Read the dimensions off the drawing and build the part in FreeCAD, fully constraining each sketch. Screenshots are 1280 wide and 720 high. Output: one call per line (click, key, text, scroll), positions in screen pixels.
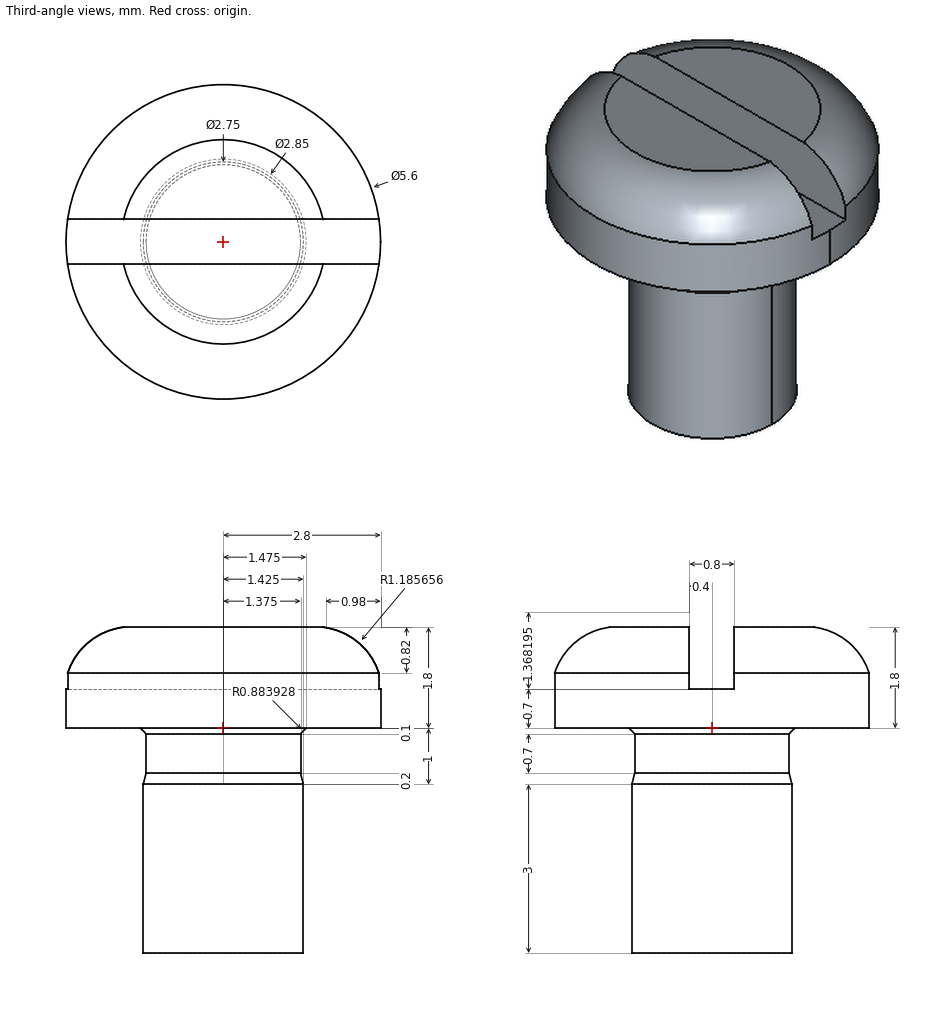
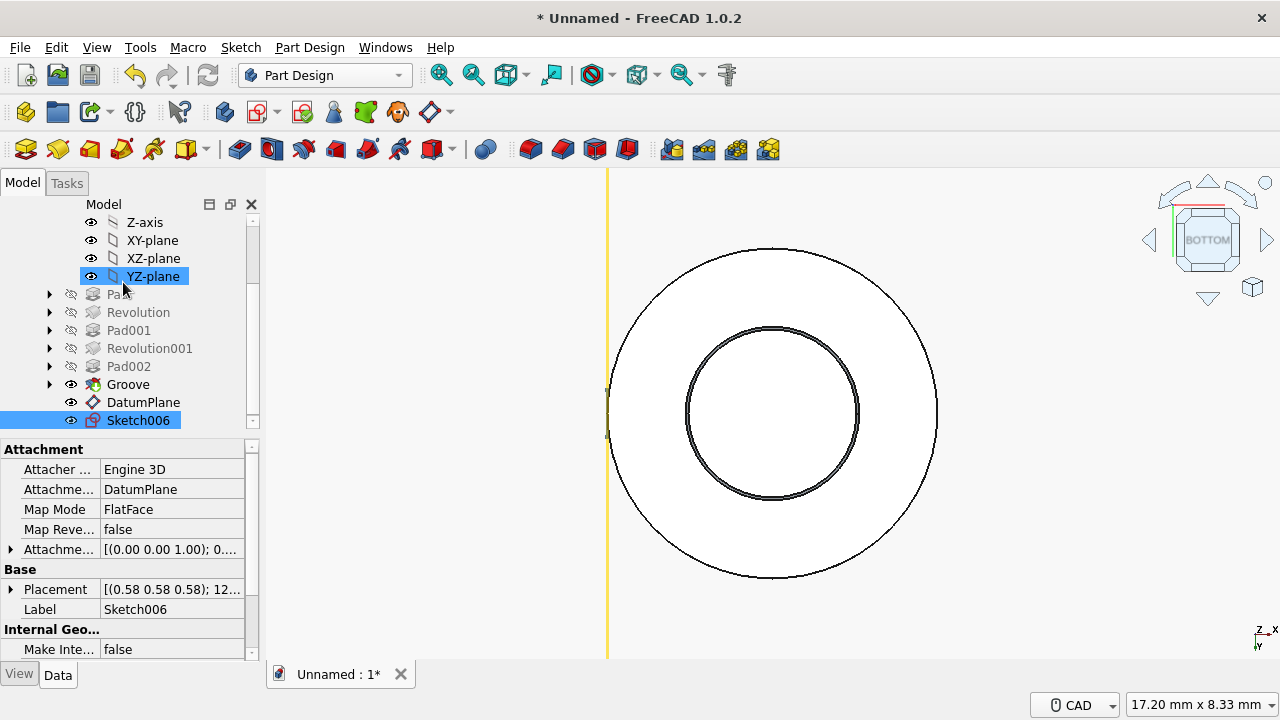
click(240, 150)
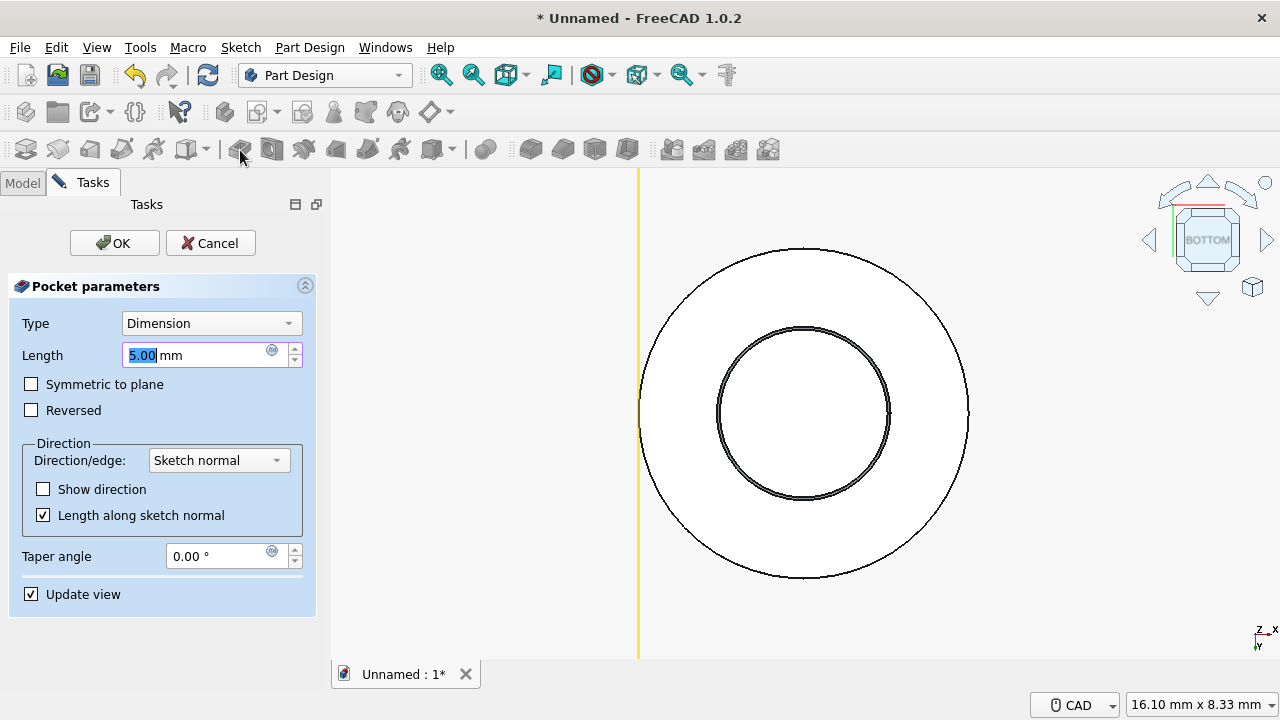
click(212, 324)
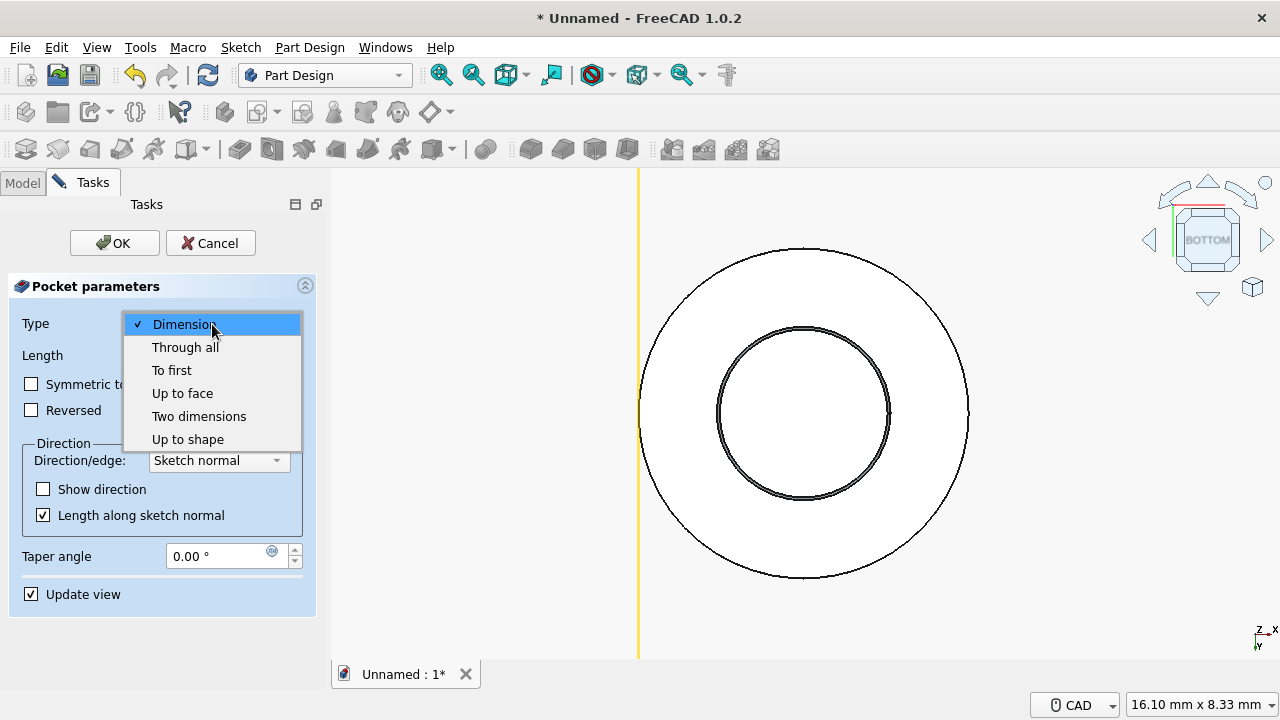
click(212, 348)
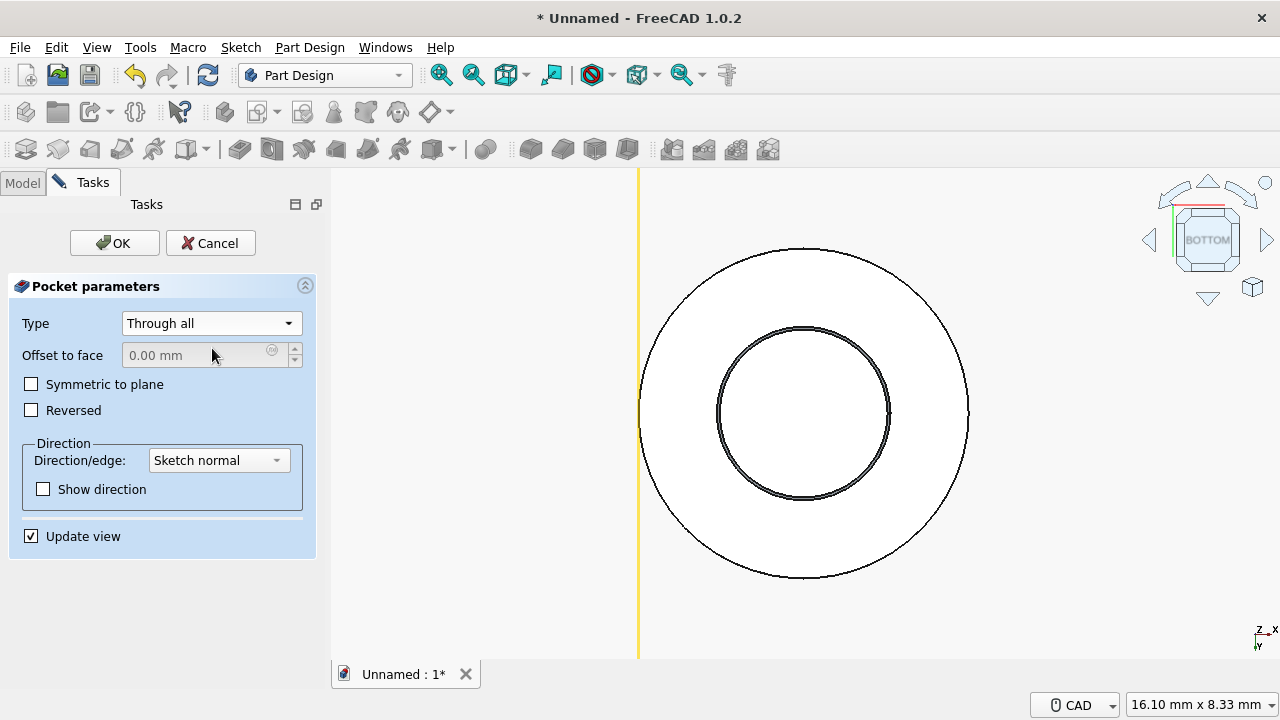
click(30, 410)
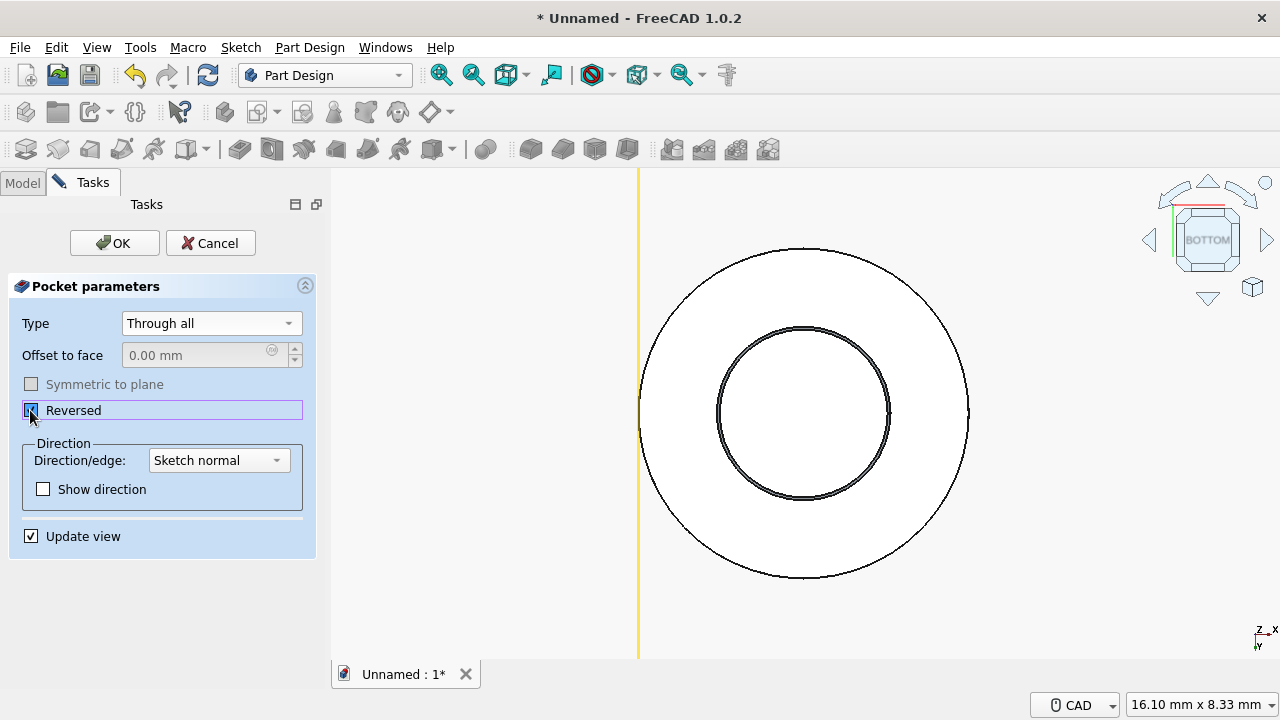
click(115, 243)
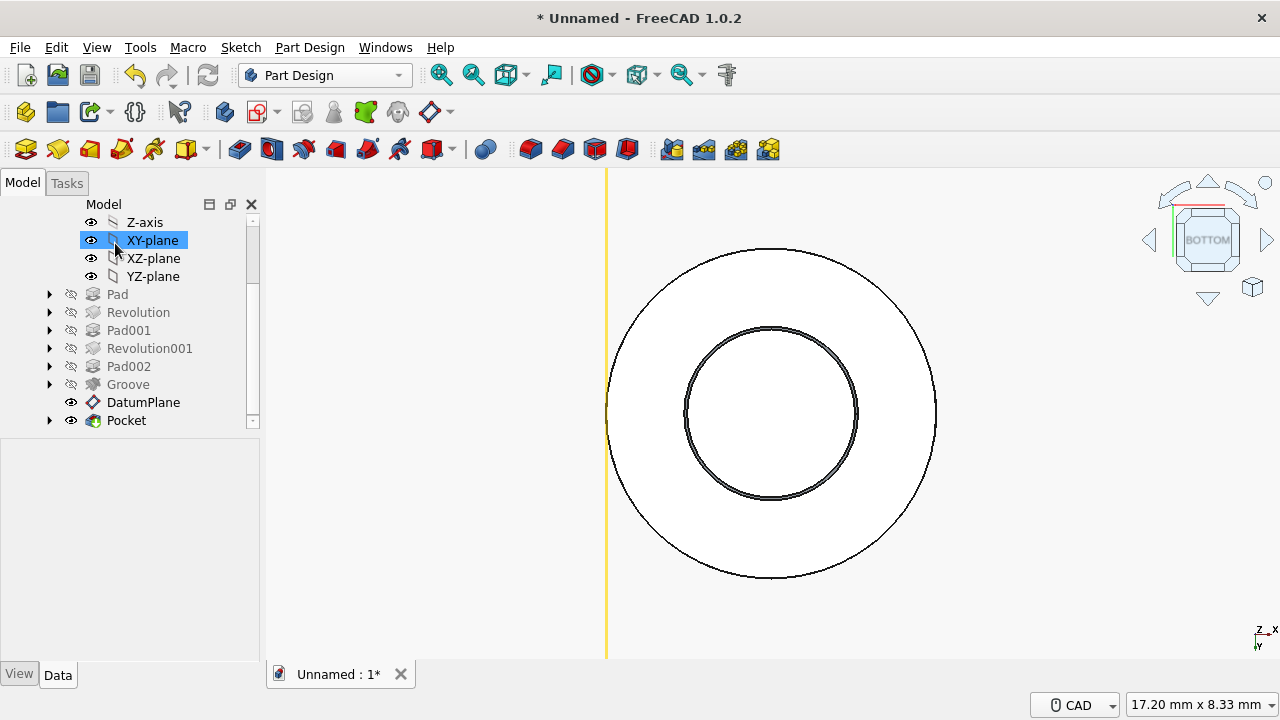
click(116, 402)
key(space)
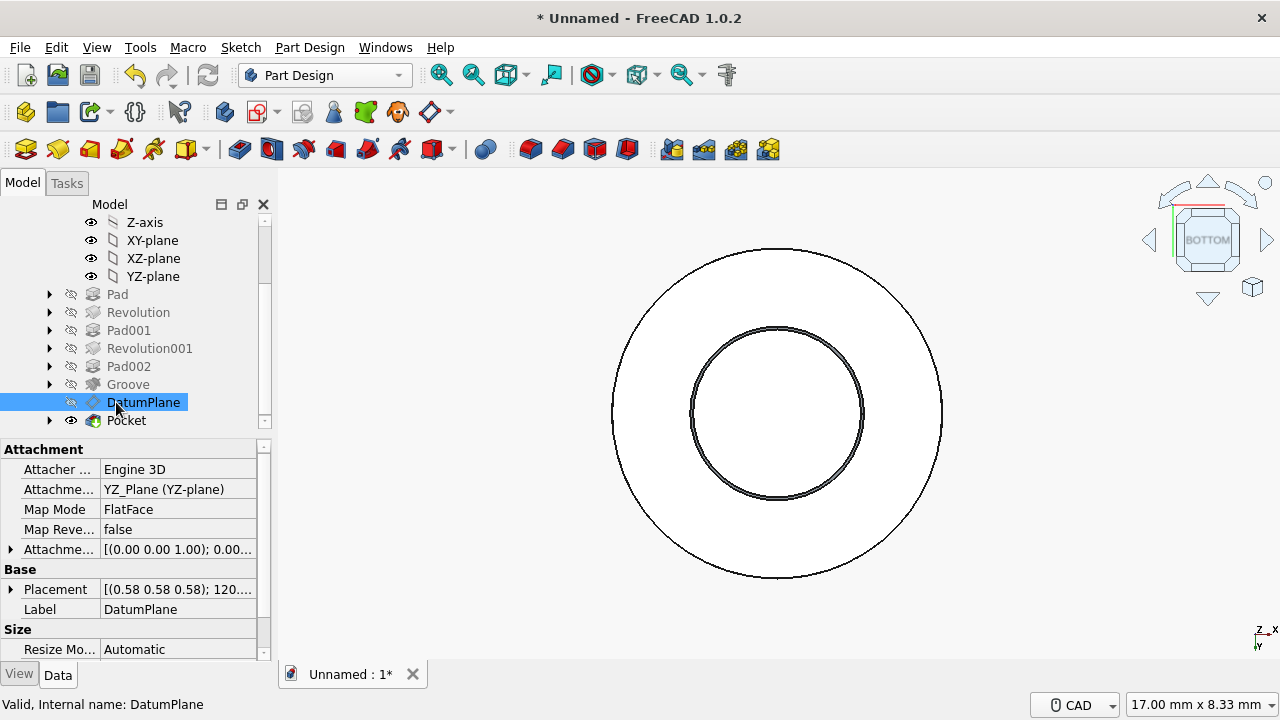
key(0)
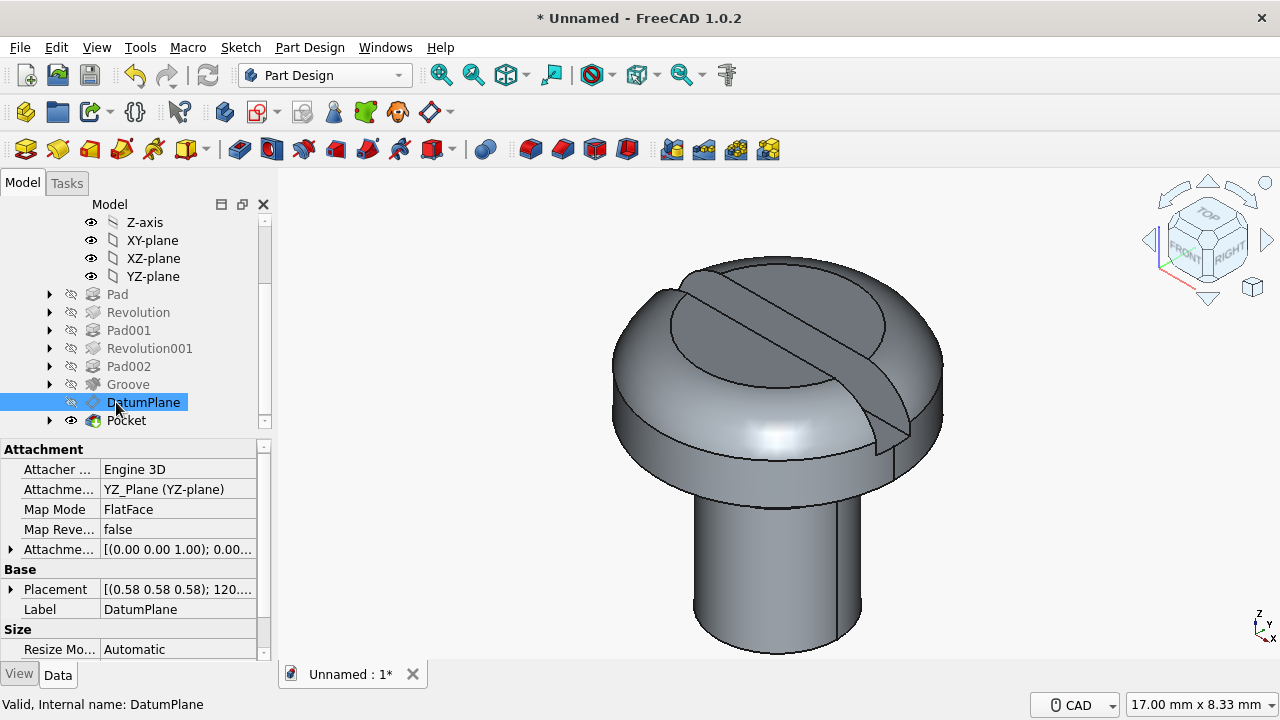
click(442, 76)